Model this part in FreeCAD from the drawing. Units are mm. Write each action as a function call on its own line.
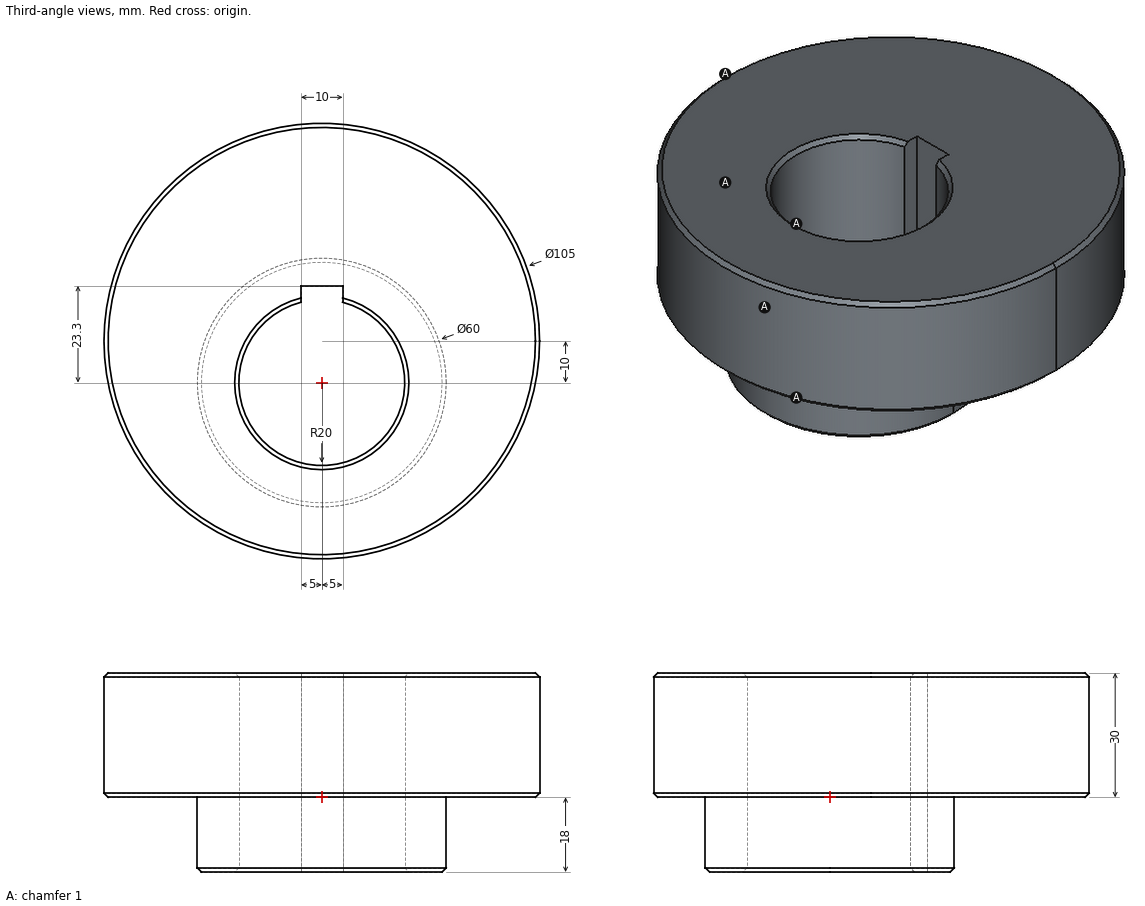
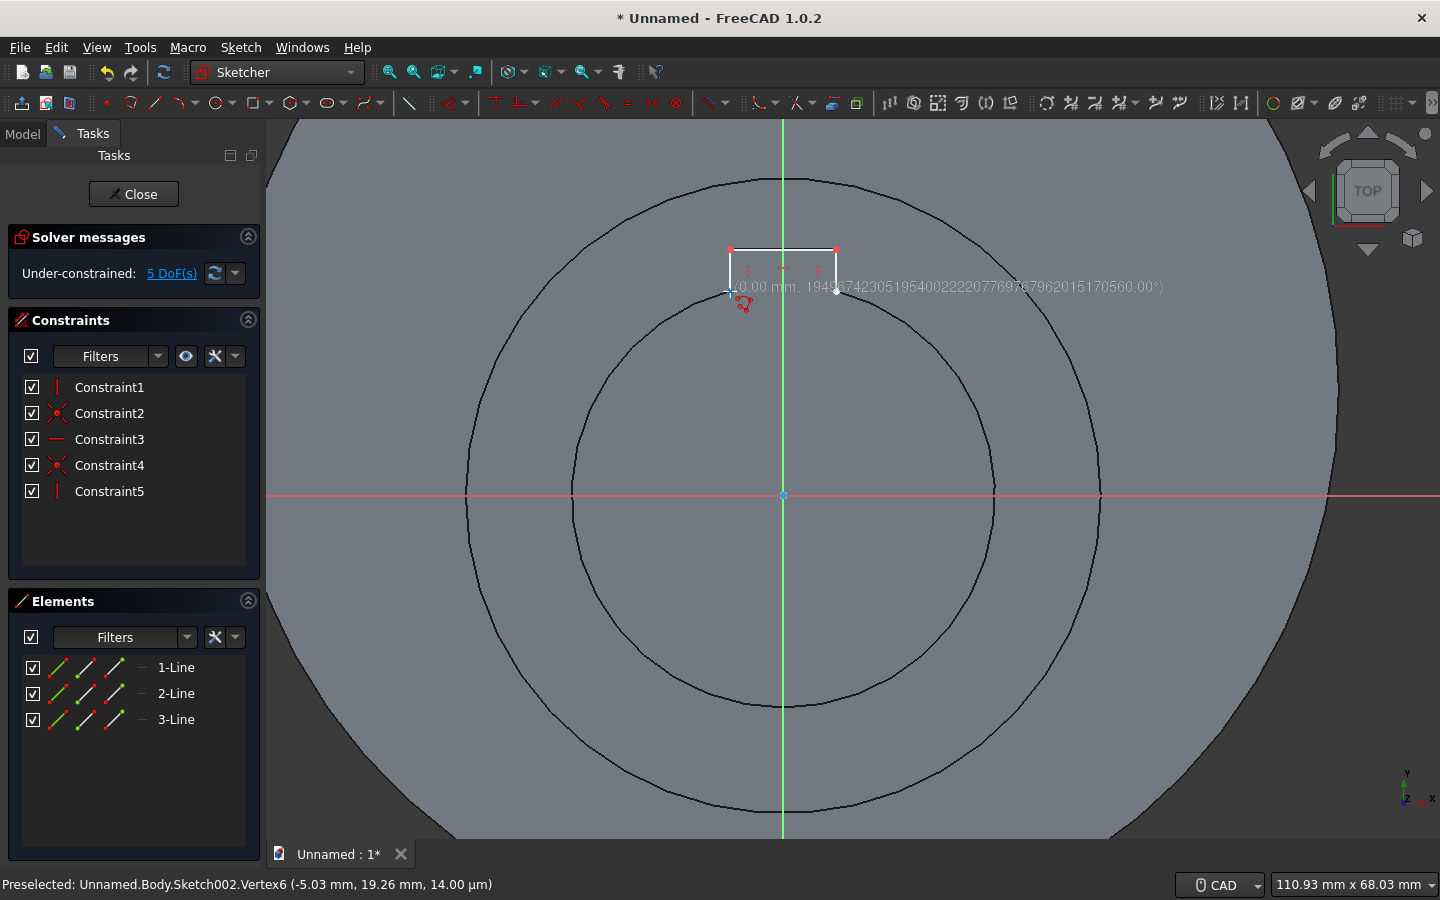
click(180, 104)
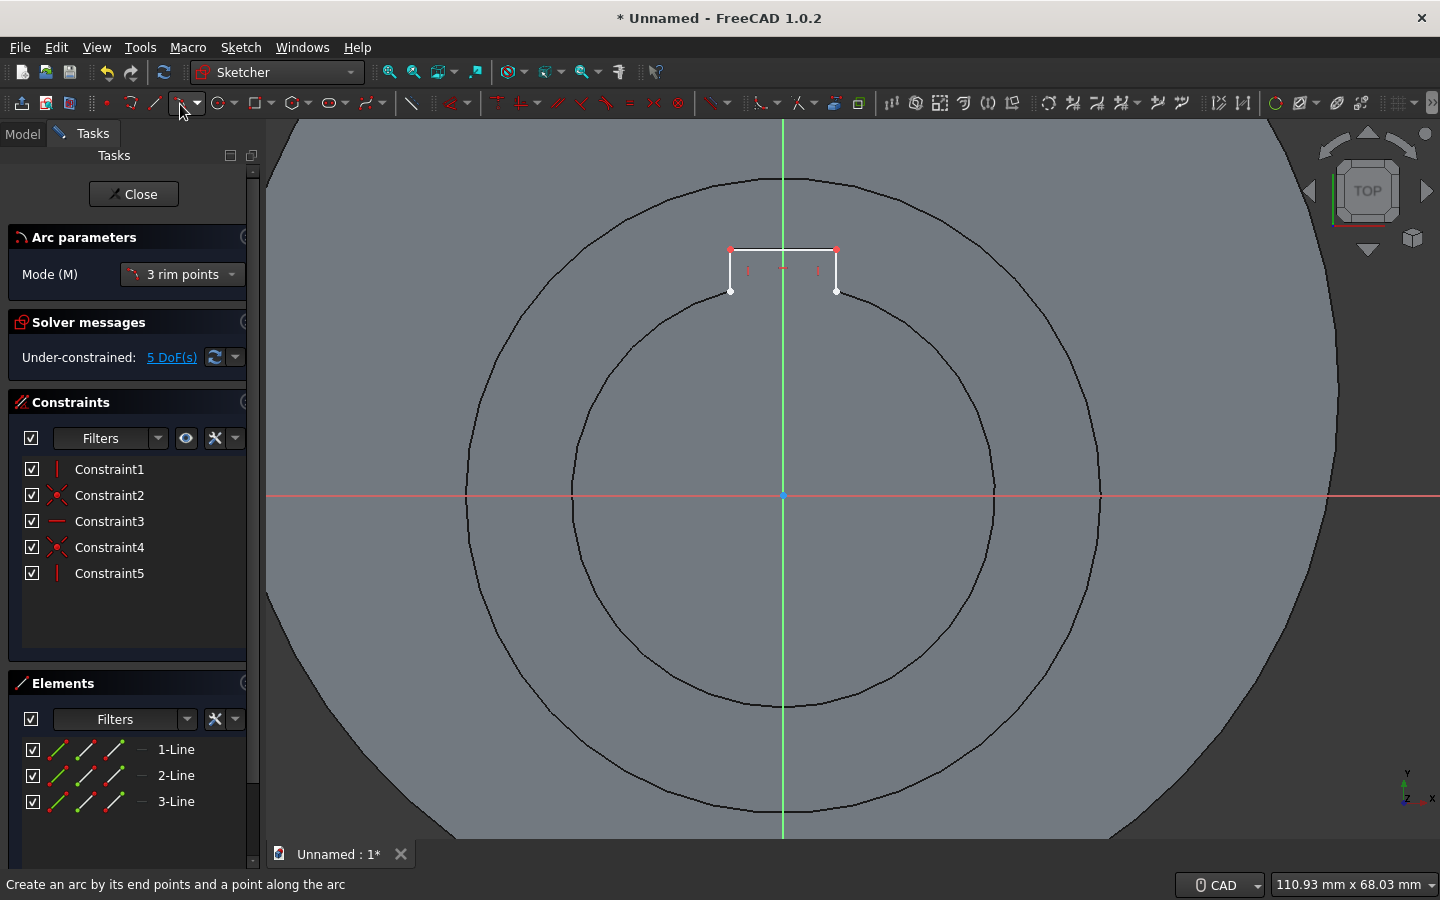
click(730, 292)
click(836, 292)
click(668, 673)
key(Escape)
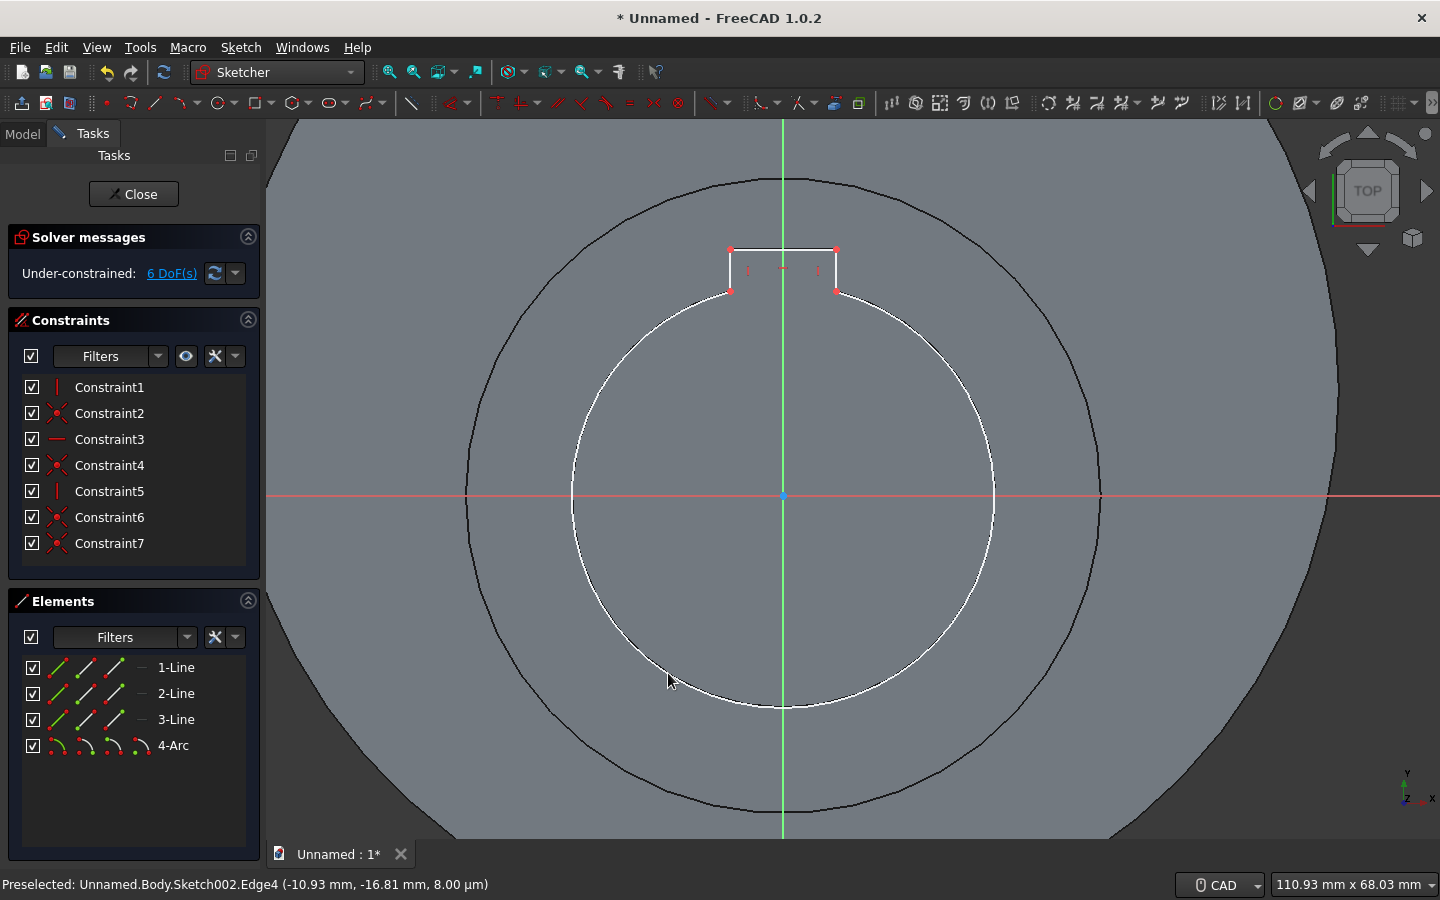
drag(773, 486, 793, 507)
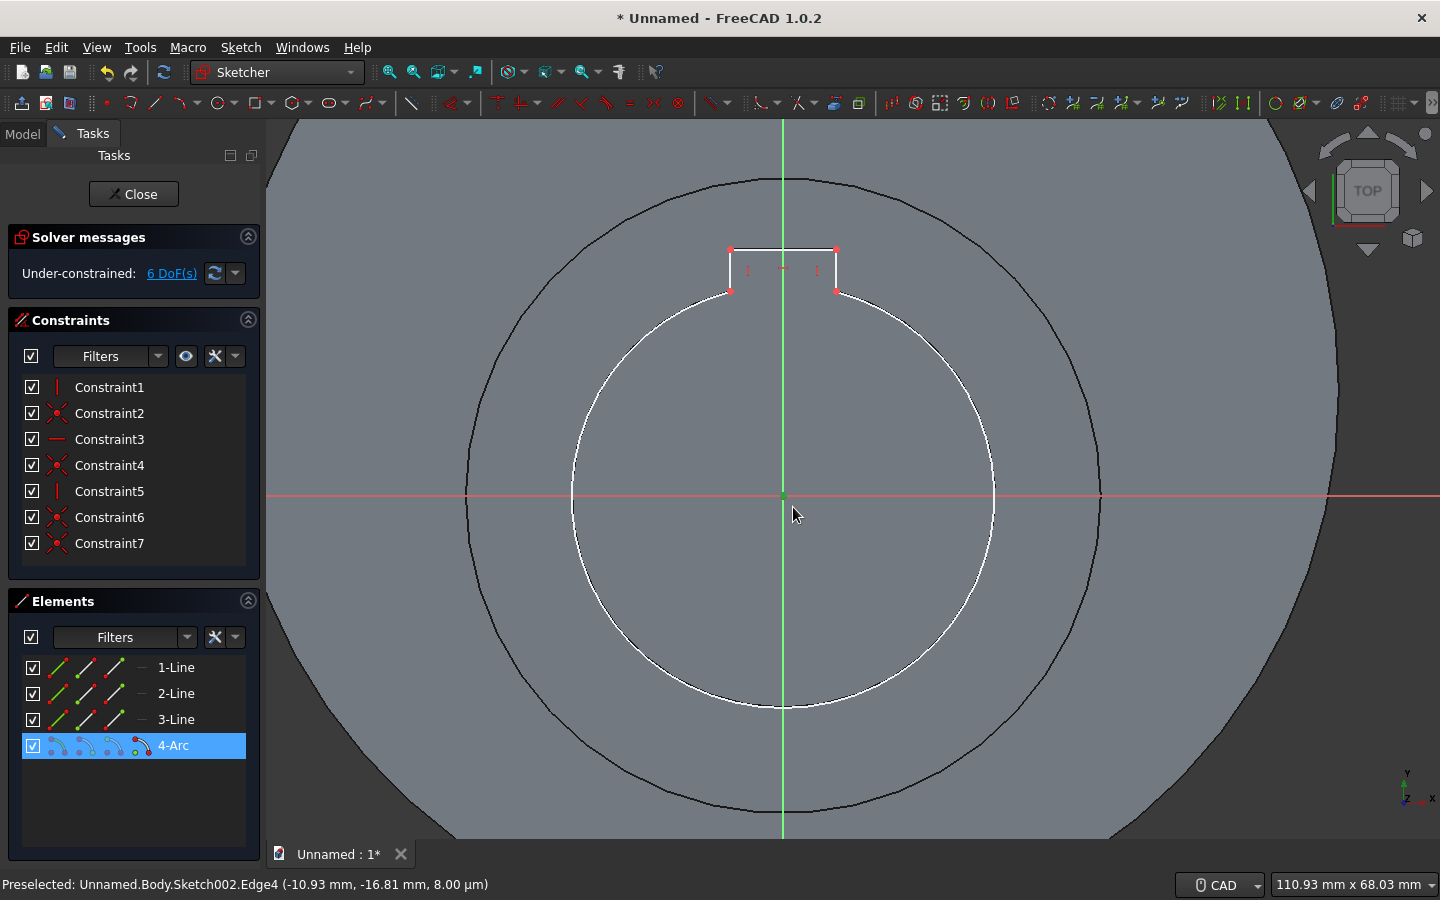
click(498, 104)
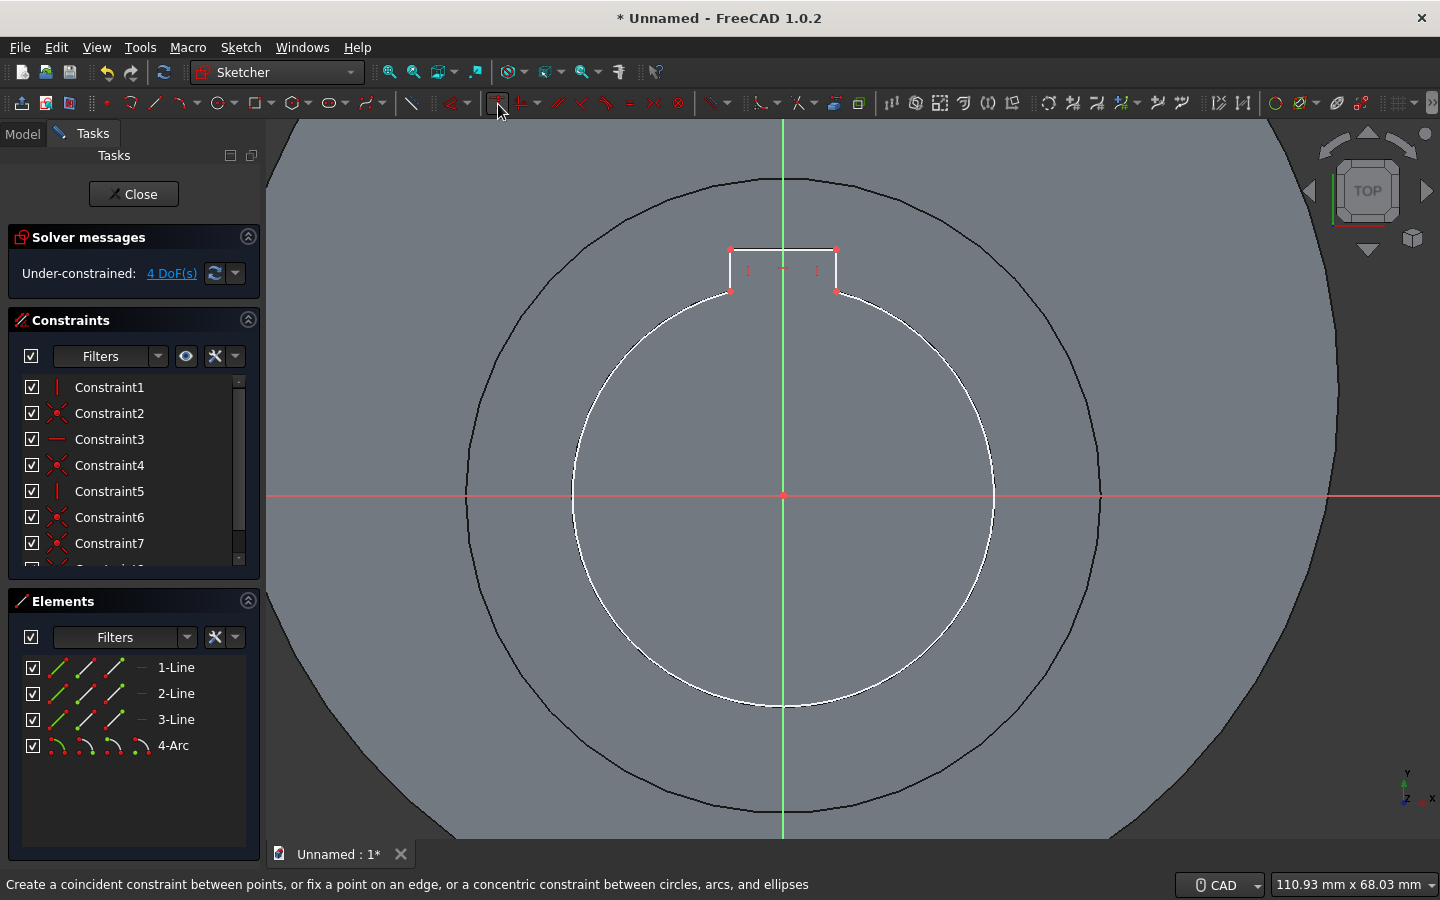
click(450, 104)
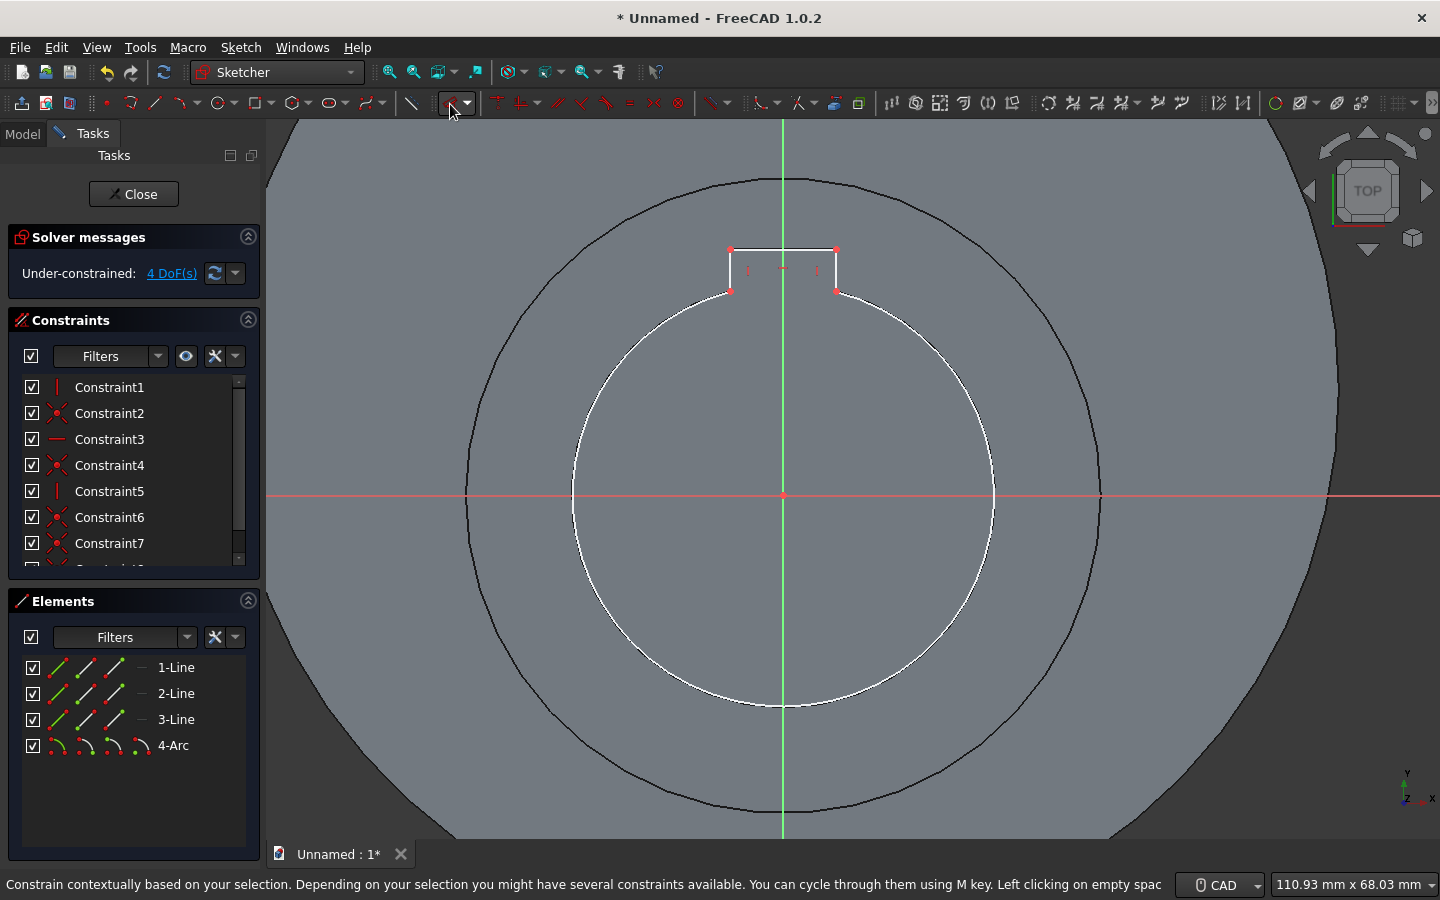
click(591, 581)
click(562, 594)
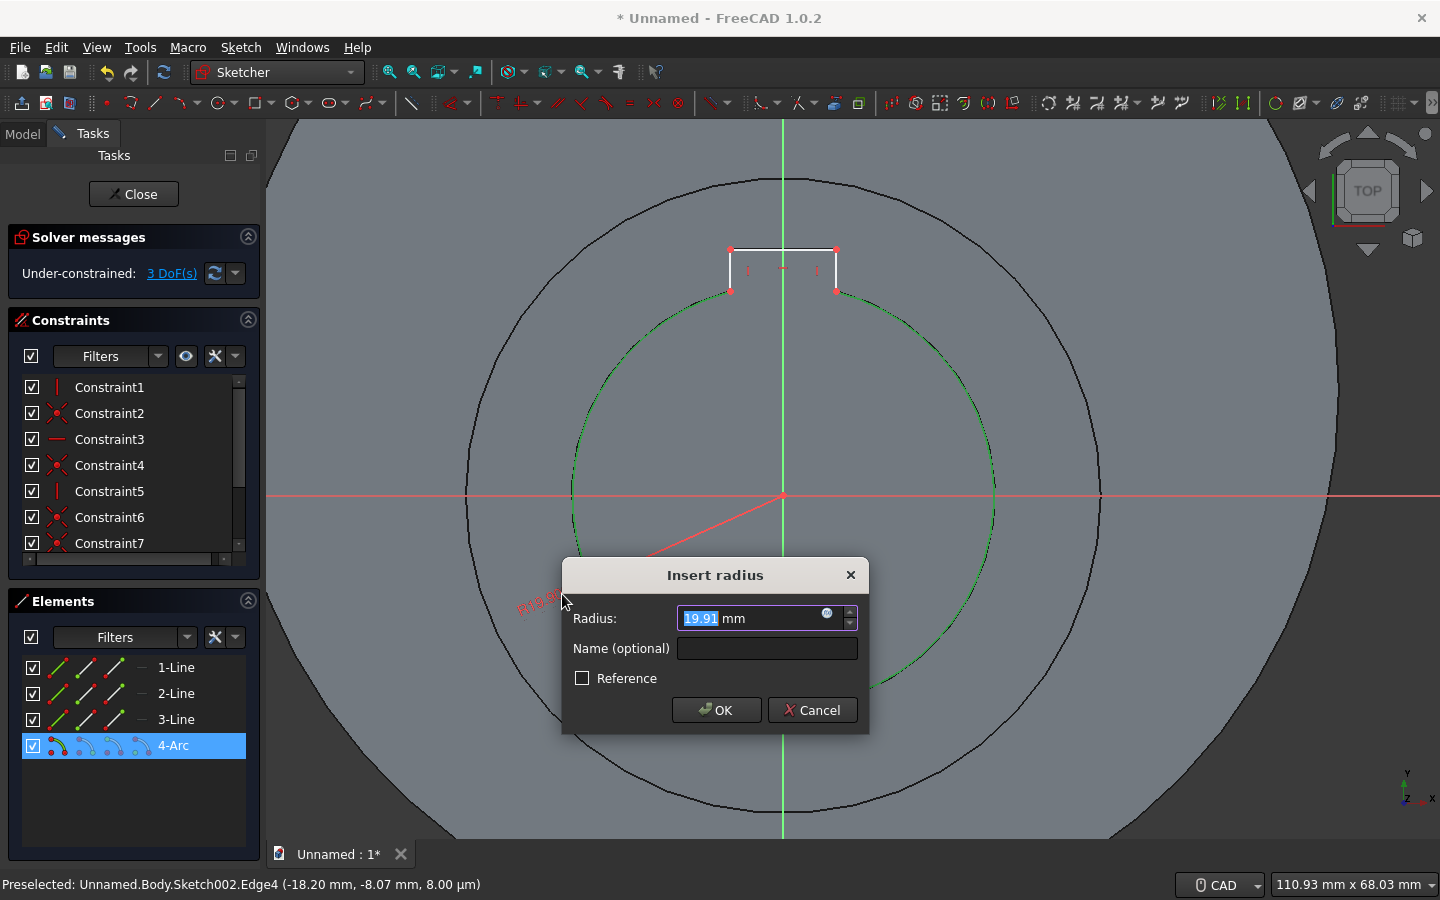
text(20)
key(Return)